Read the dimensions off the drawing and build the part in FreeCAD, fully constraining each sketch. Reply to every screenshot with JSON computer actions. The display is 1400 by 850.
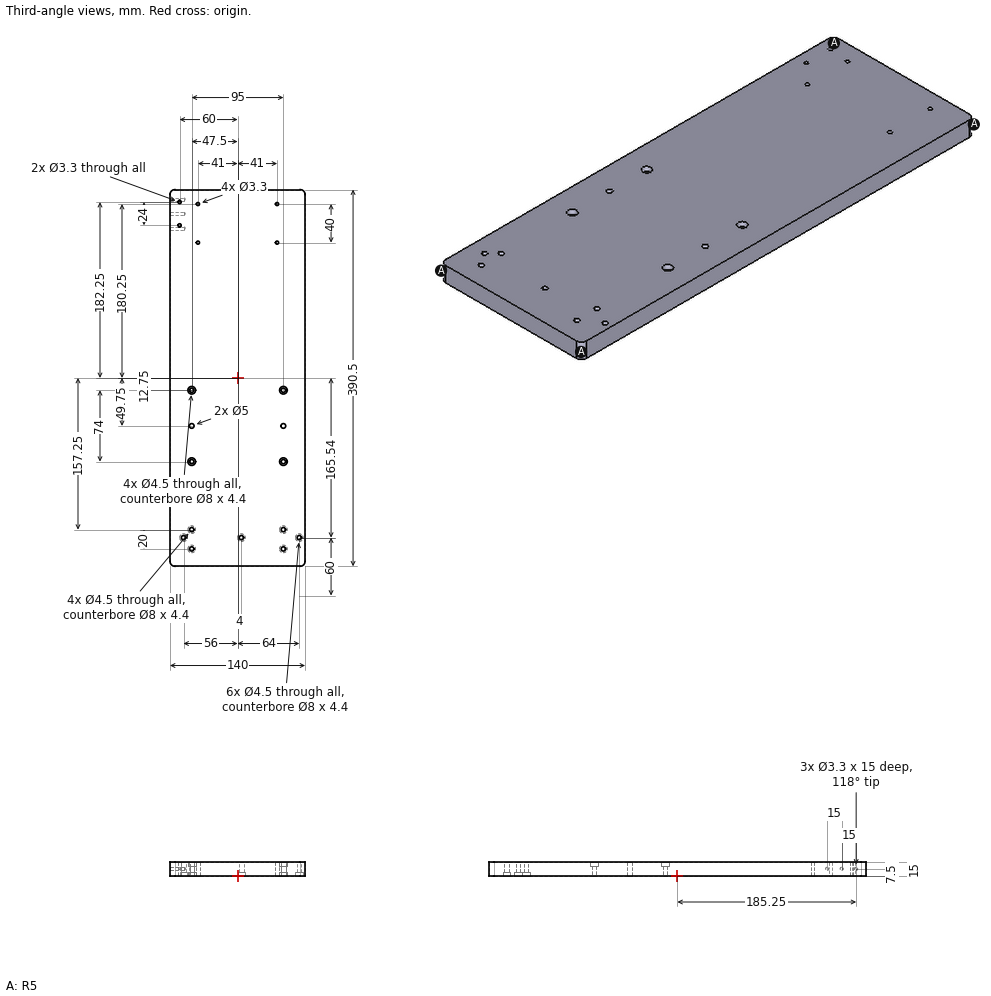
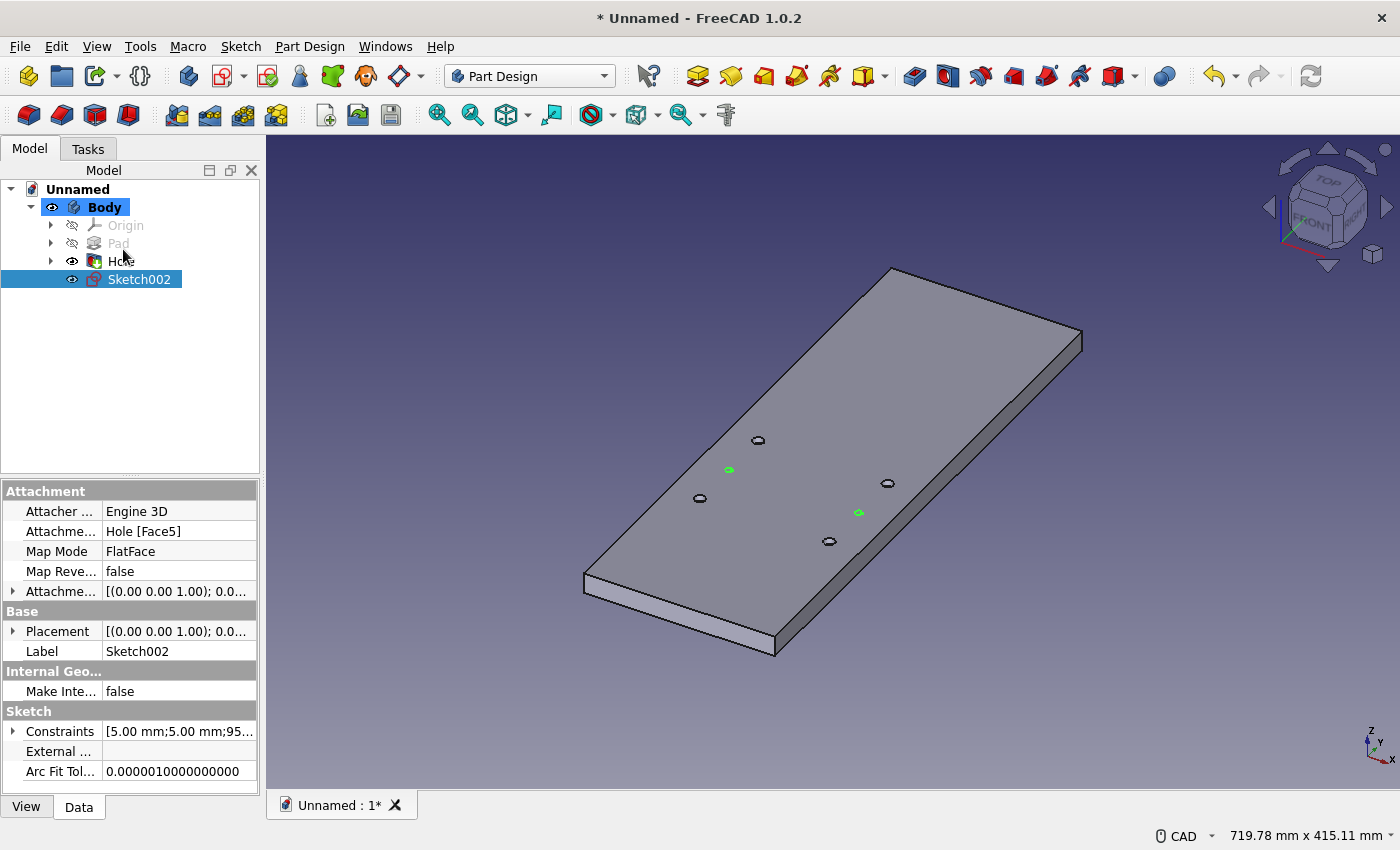
{"action": "left_click", "coordinate": [915, 76]}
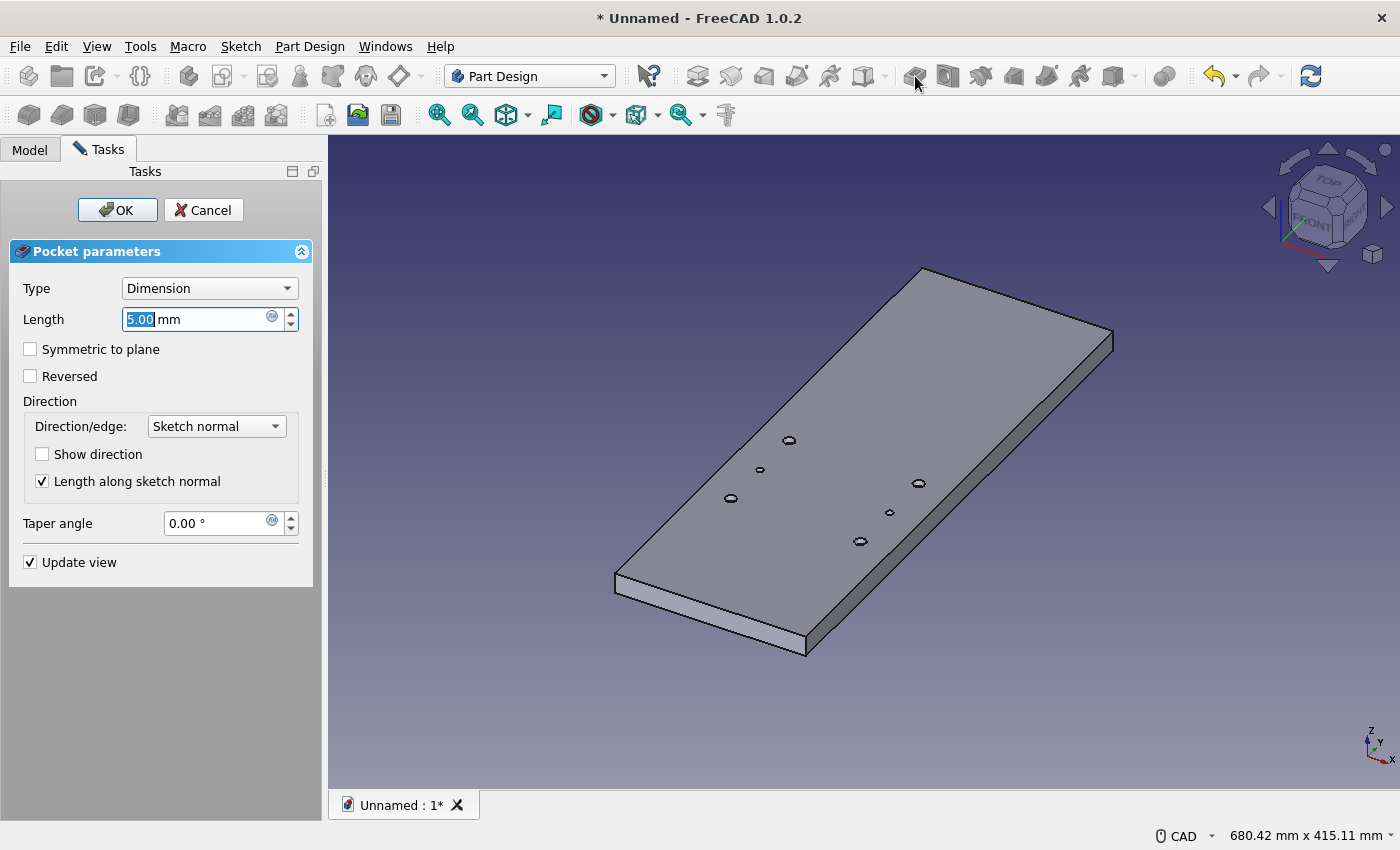
{"action": "left_click", "coordinate": [210, 288]}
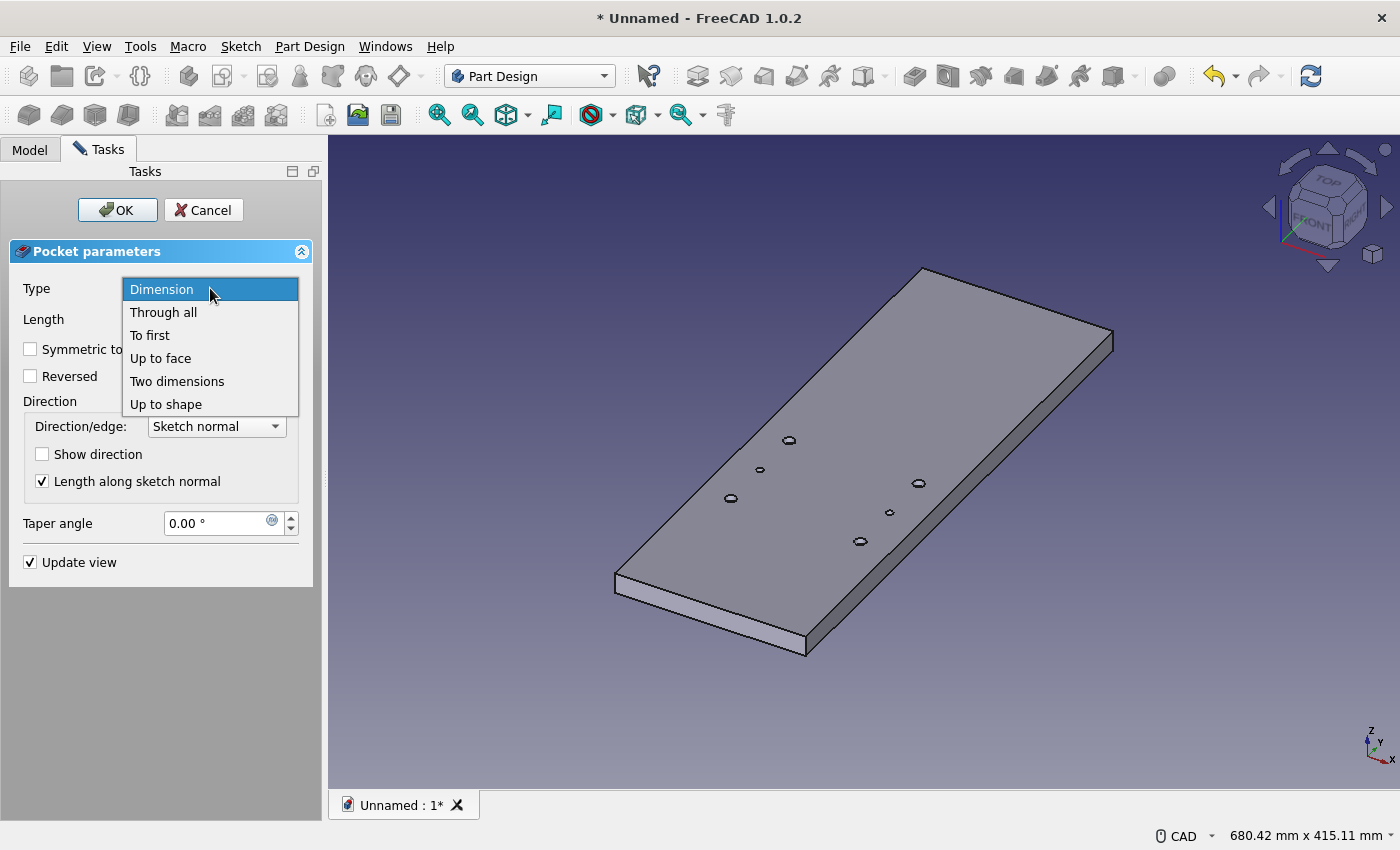
{"action": "left_click", "coordinate": [208, 312]}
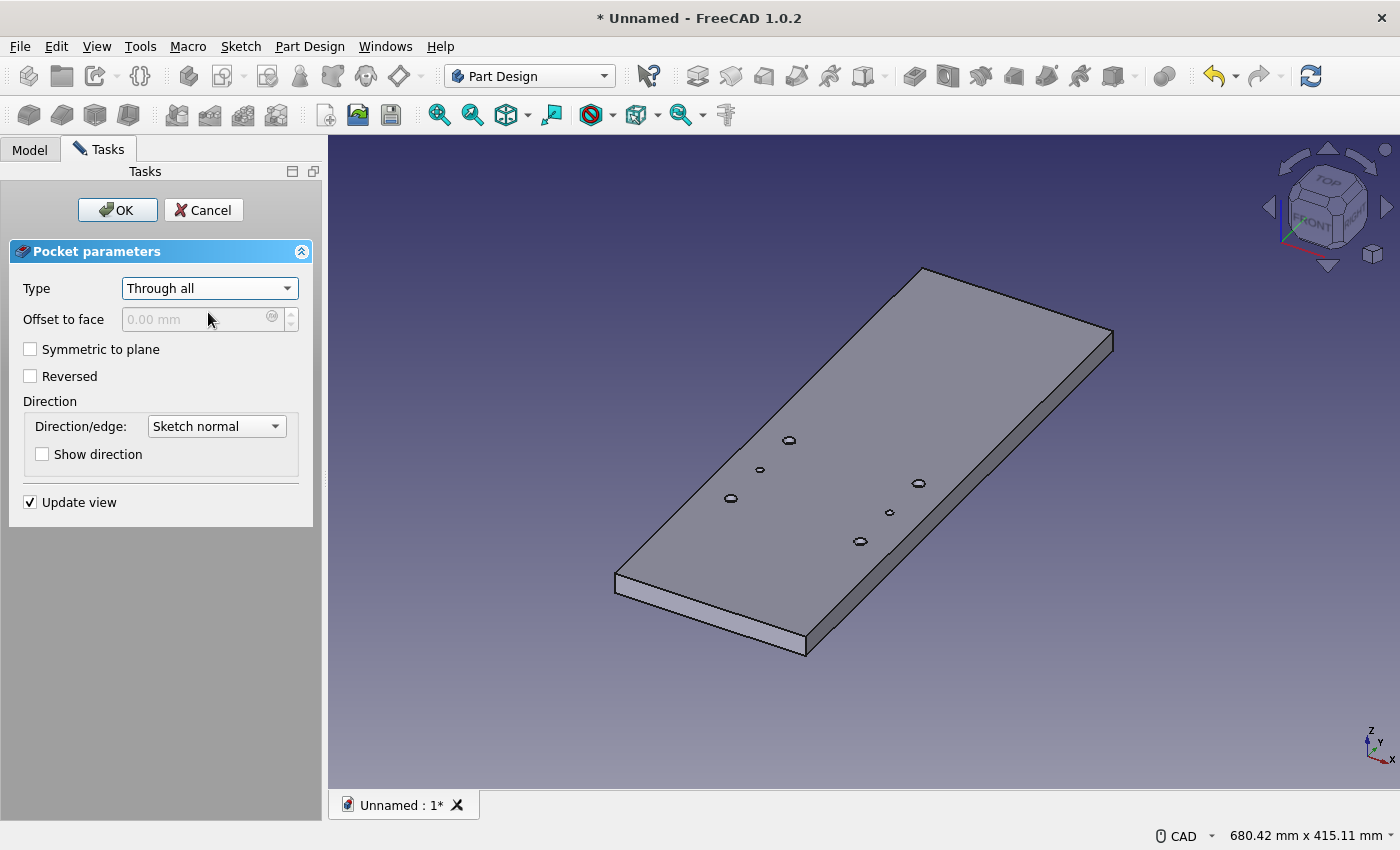
{"action": "left_click", "coordinate": [118, 210]}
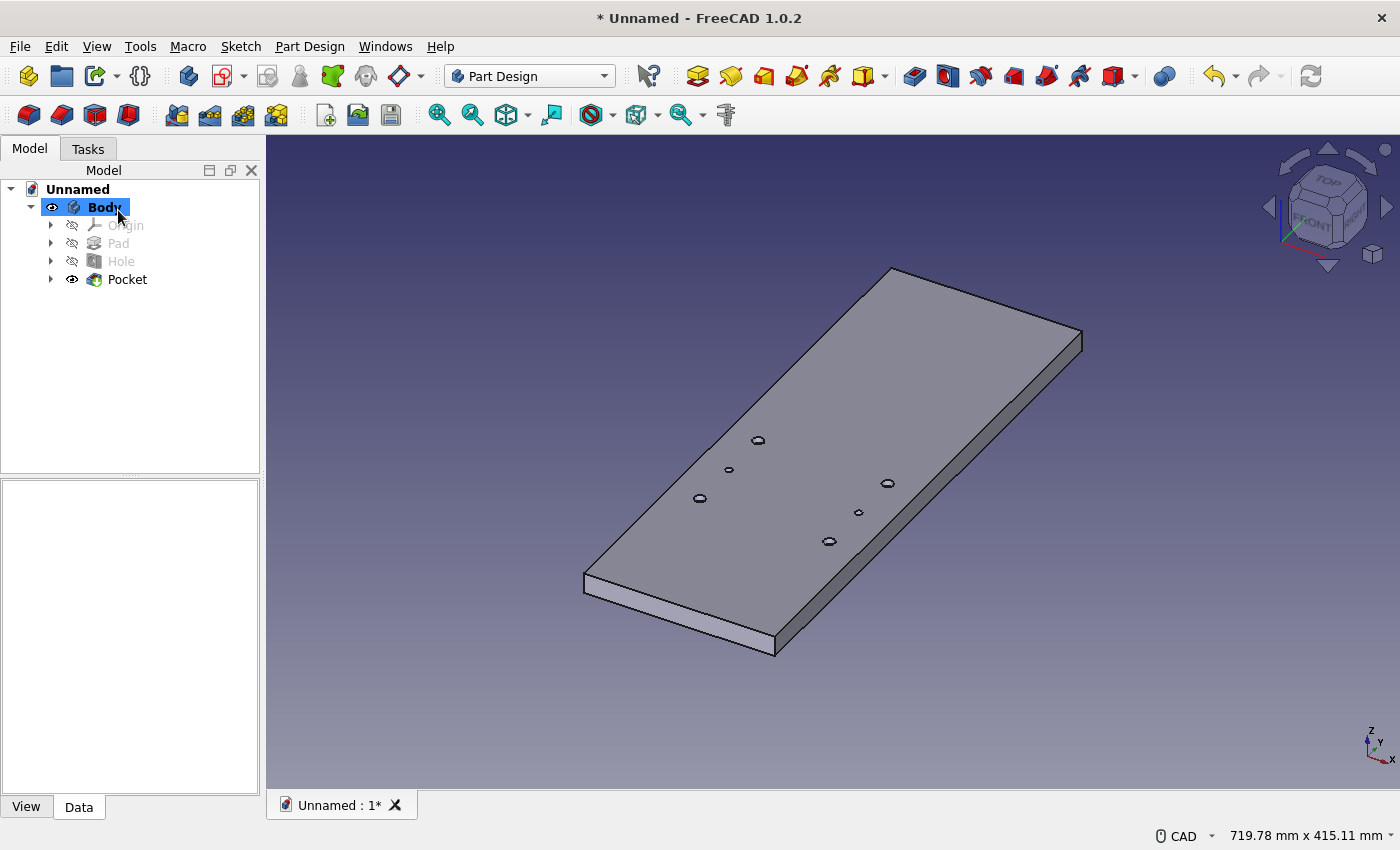
{"action": "left_click", "coordinate": [775, 645]}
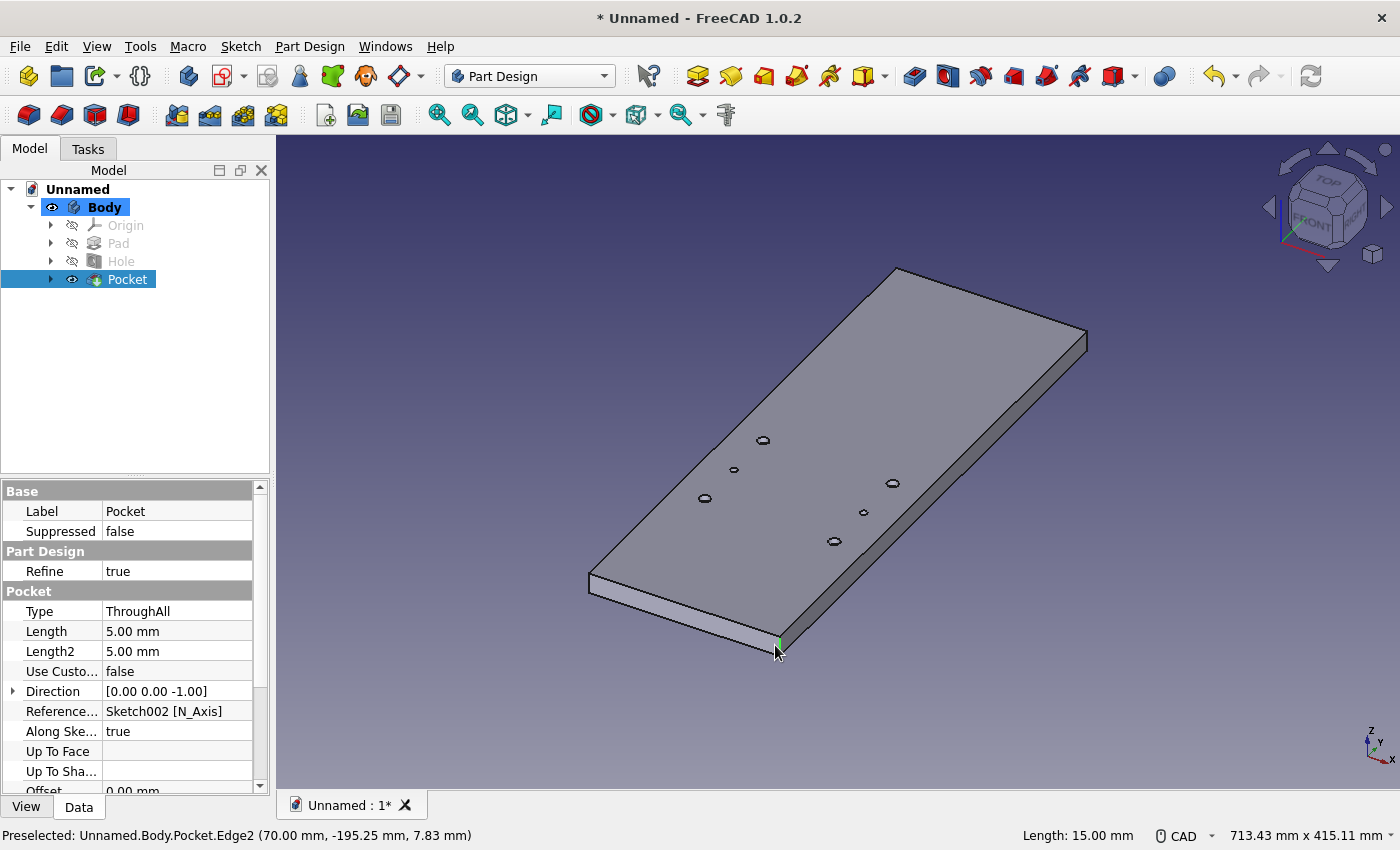
{"action": "key", "text": "0"}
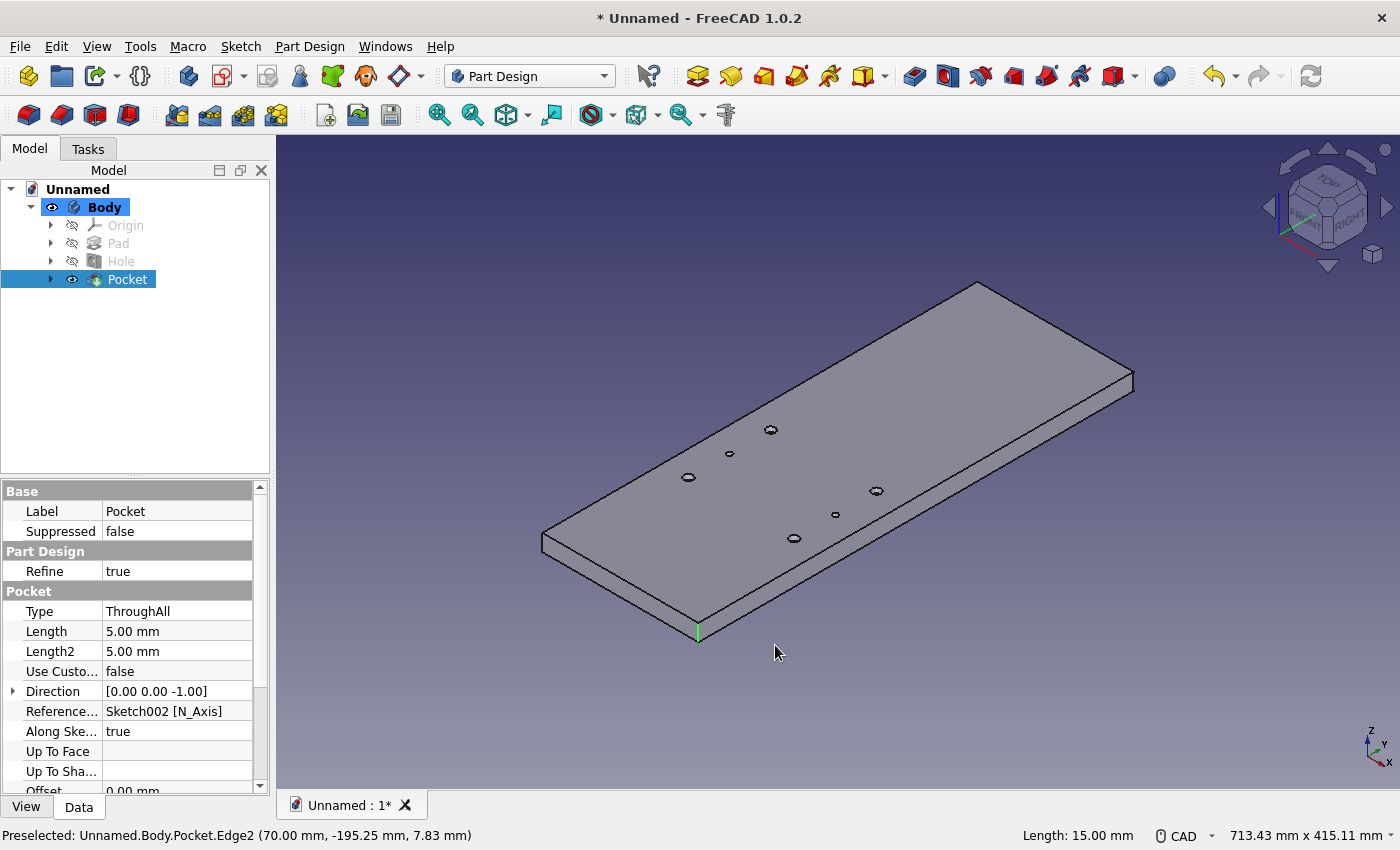
{"action": "key", "text": "2"}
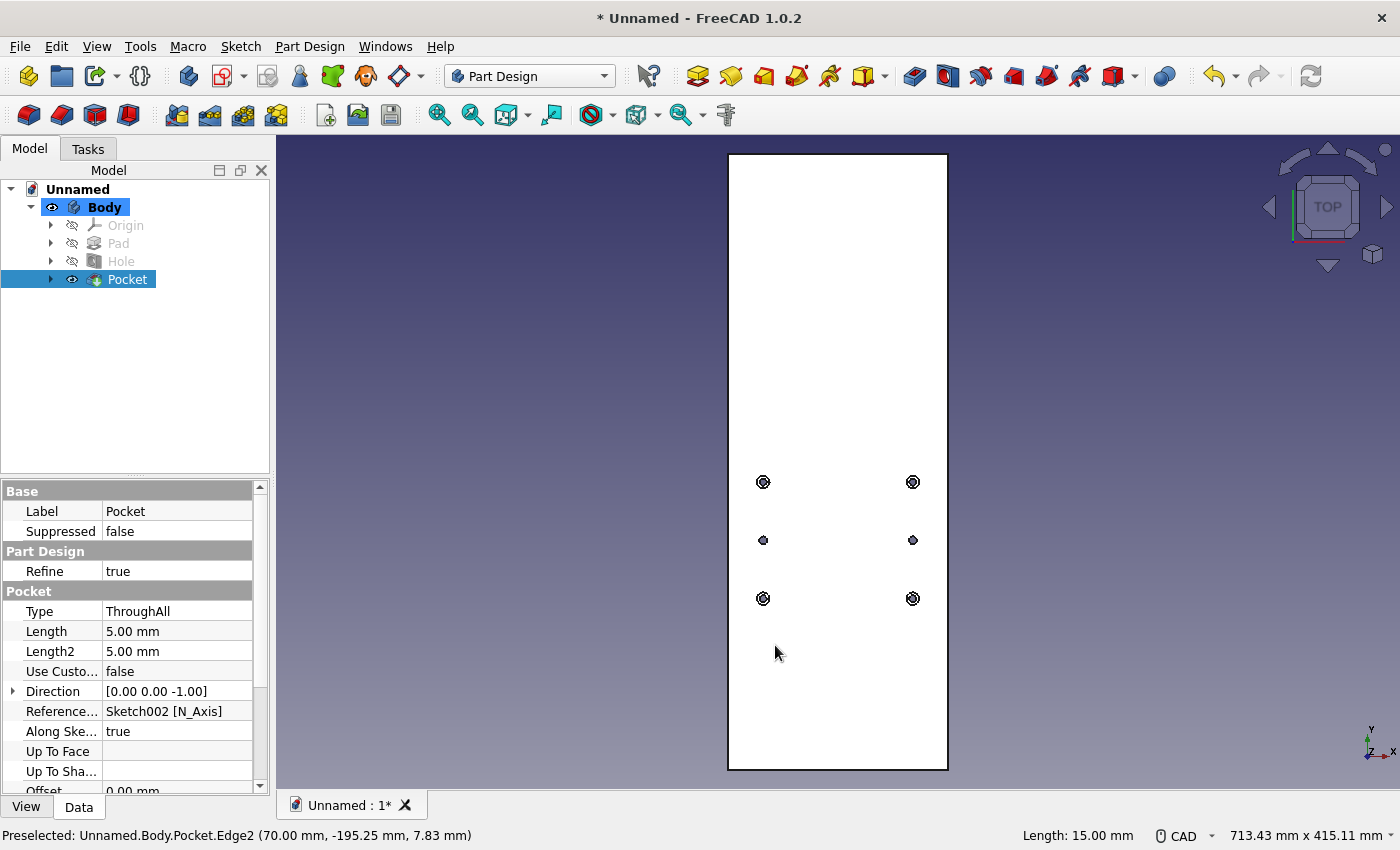
{"action": "key", "text": "1"}